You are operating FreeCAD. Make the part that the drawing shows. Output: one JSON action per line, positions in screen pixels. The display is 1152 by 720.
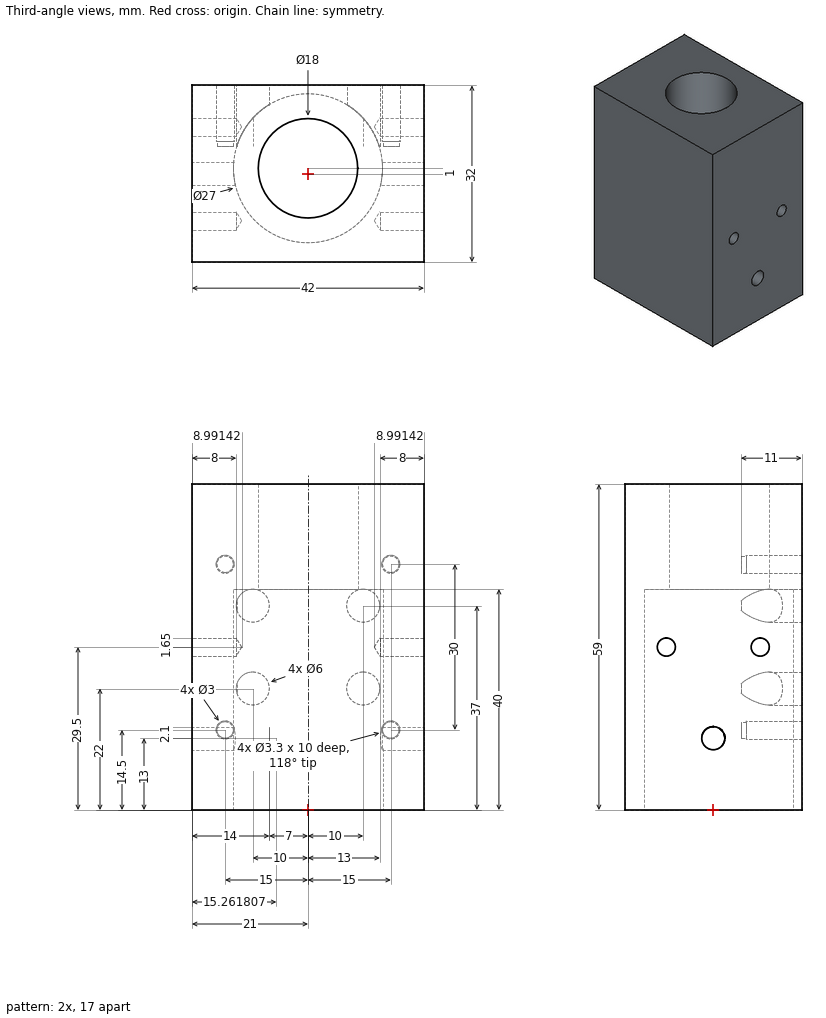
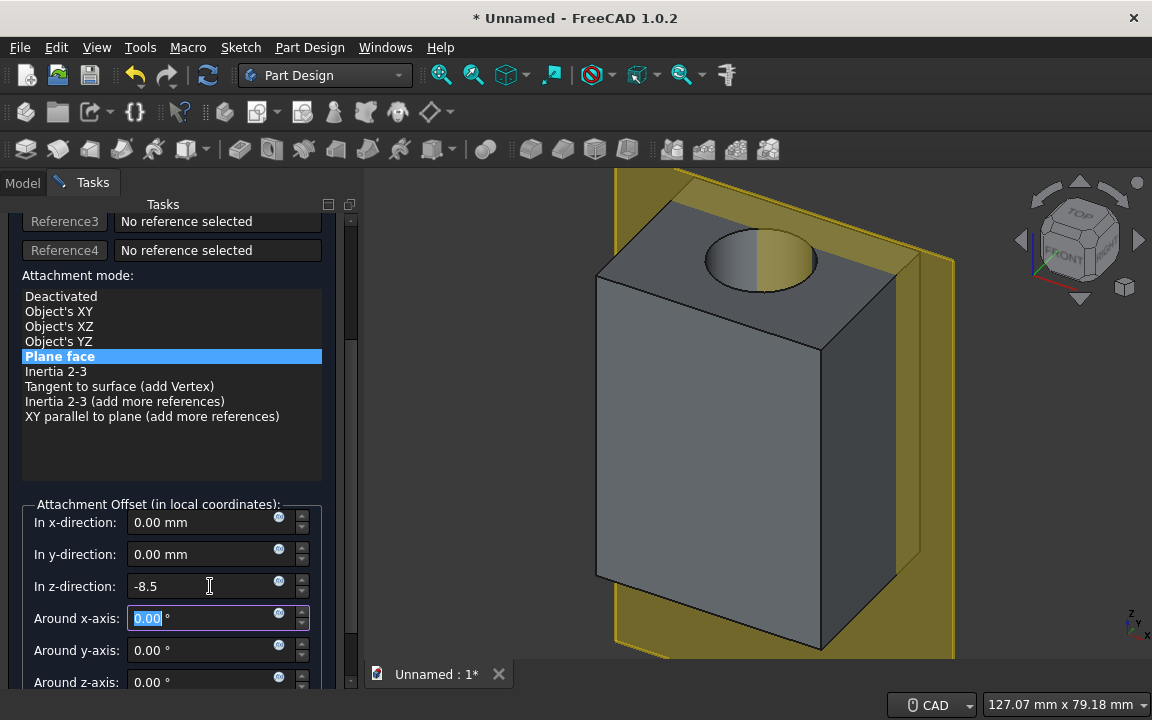
{"action": "scroll", "coordinate": [351, 451], "scroll_direction": "up", "scroll_amount": 4}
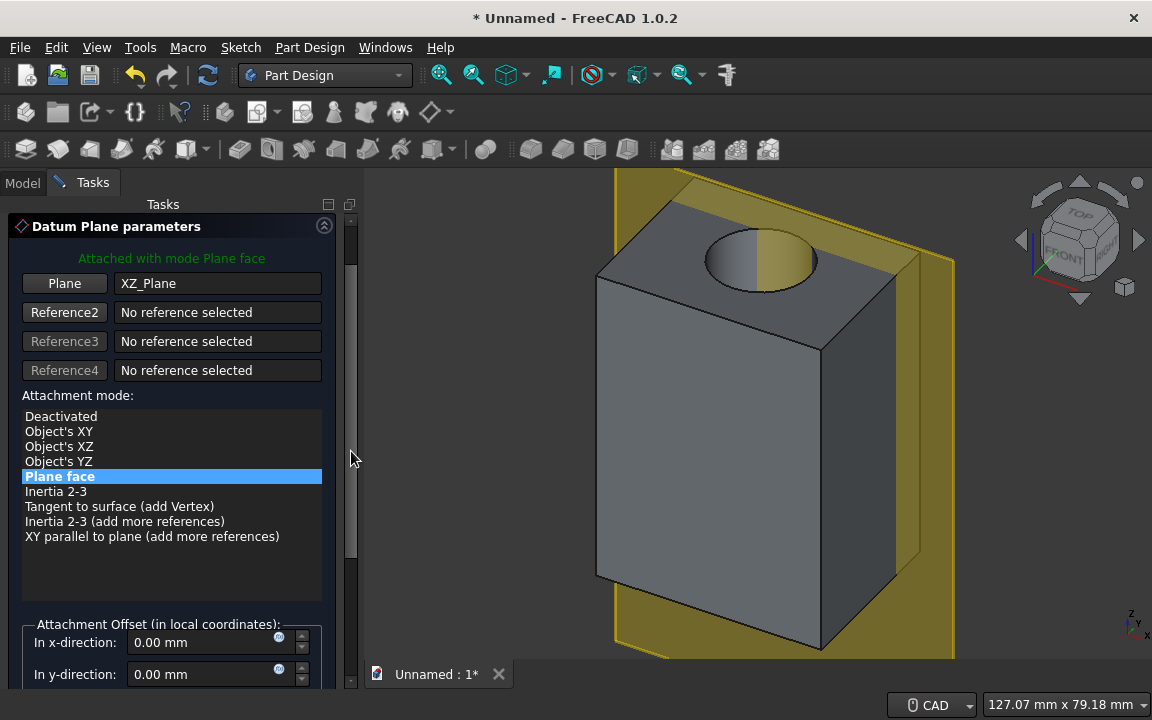
{"action": "left_click", "coordinate": [124, 243]}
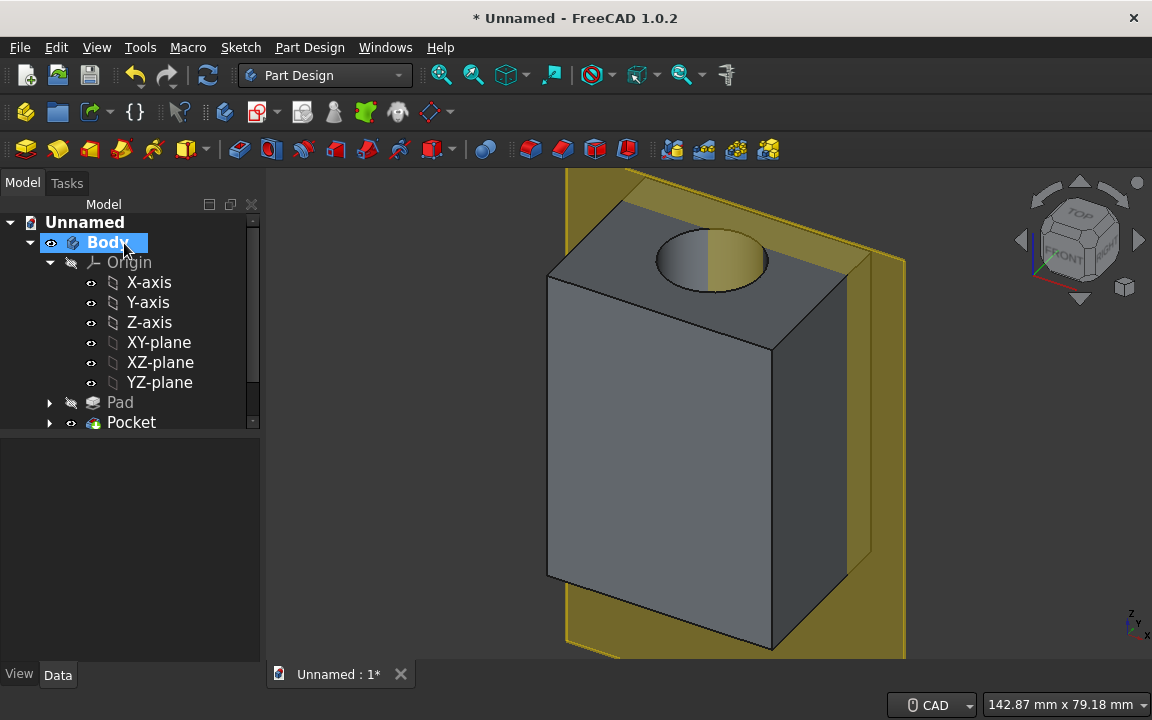
{"action": "scroll", "coordinate": [100, 318], "scroll_direction": "down", "scroll_amount": 3}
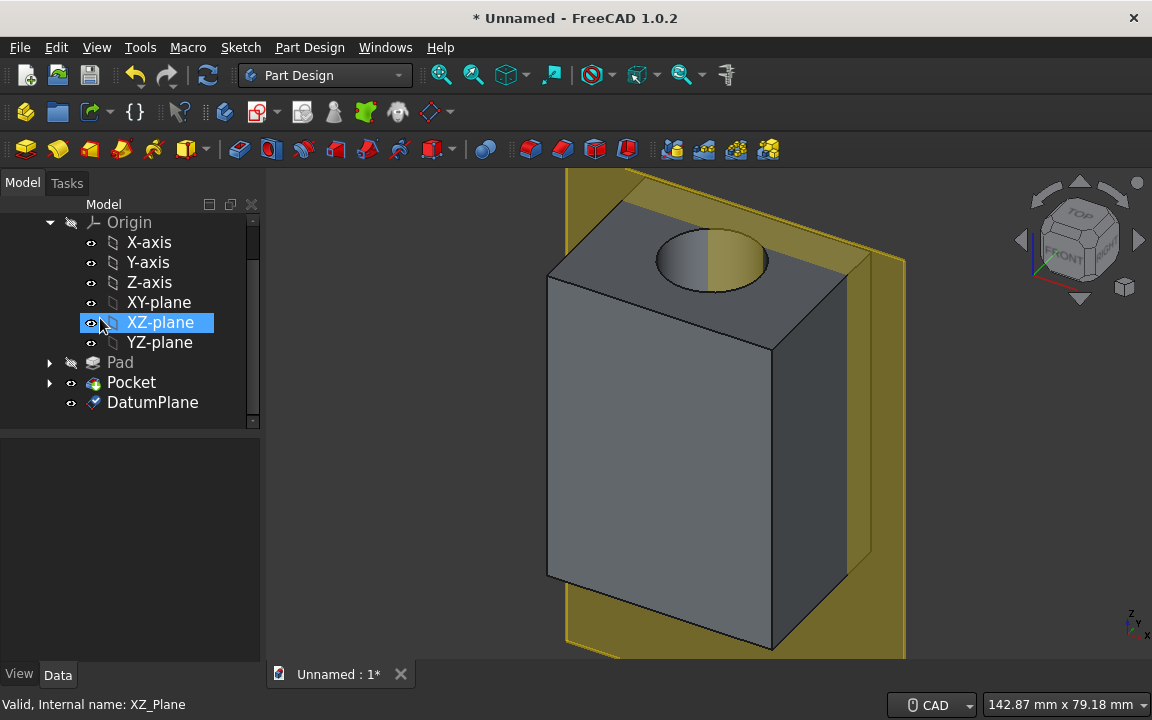
{"action": "left_click", "coordinate": [116, 403]}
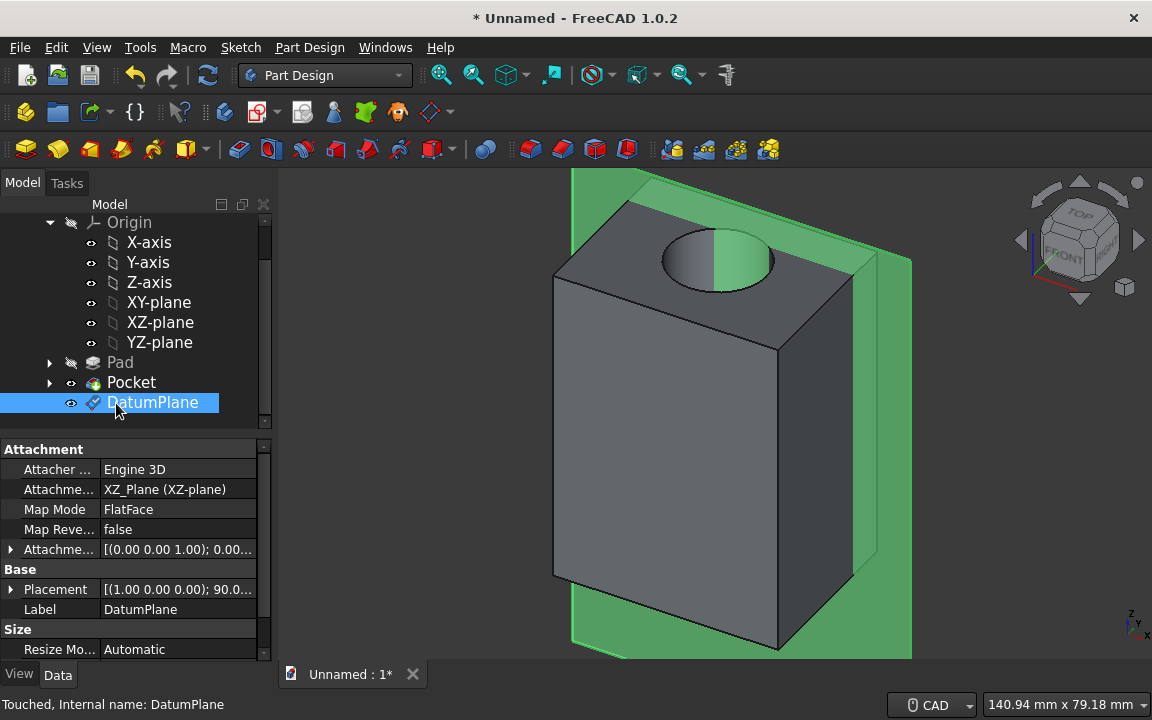
{"action": "left_click", "coordinate": [258, 112]}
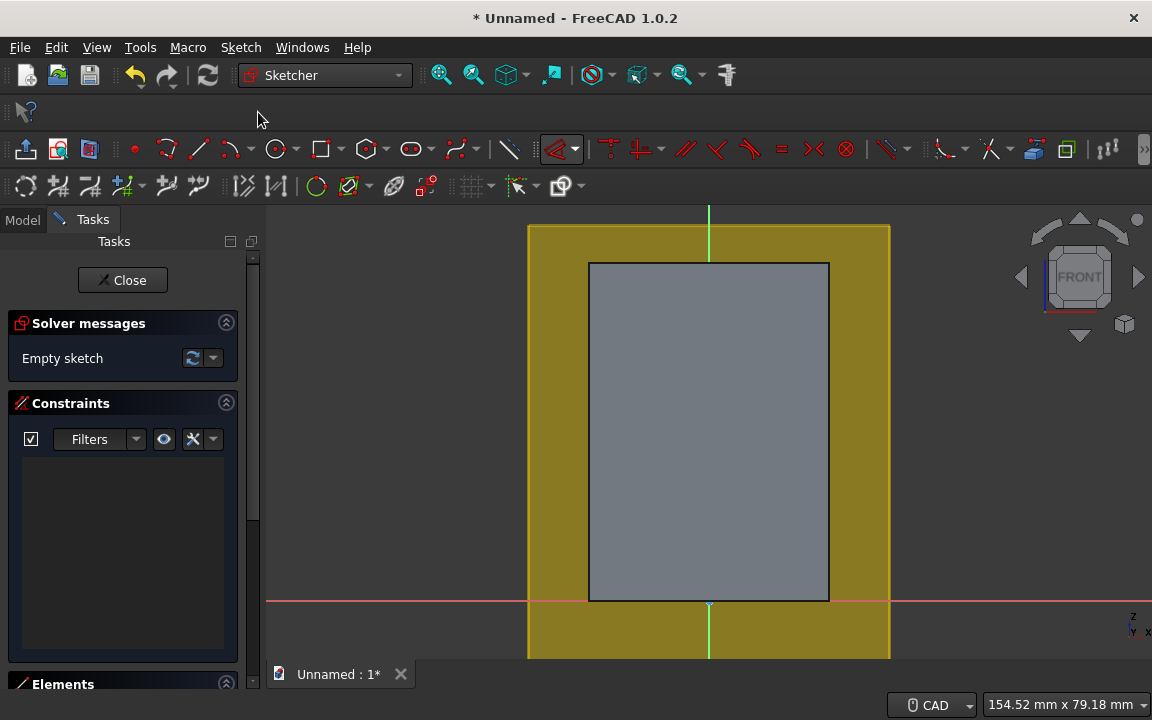
{"action": "key", "text": "q s"}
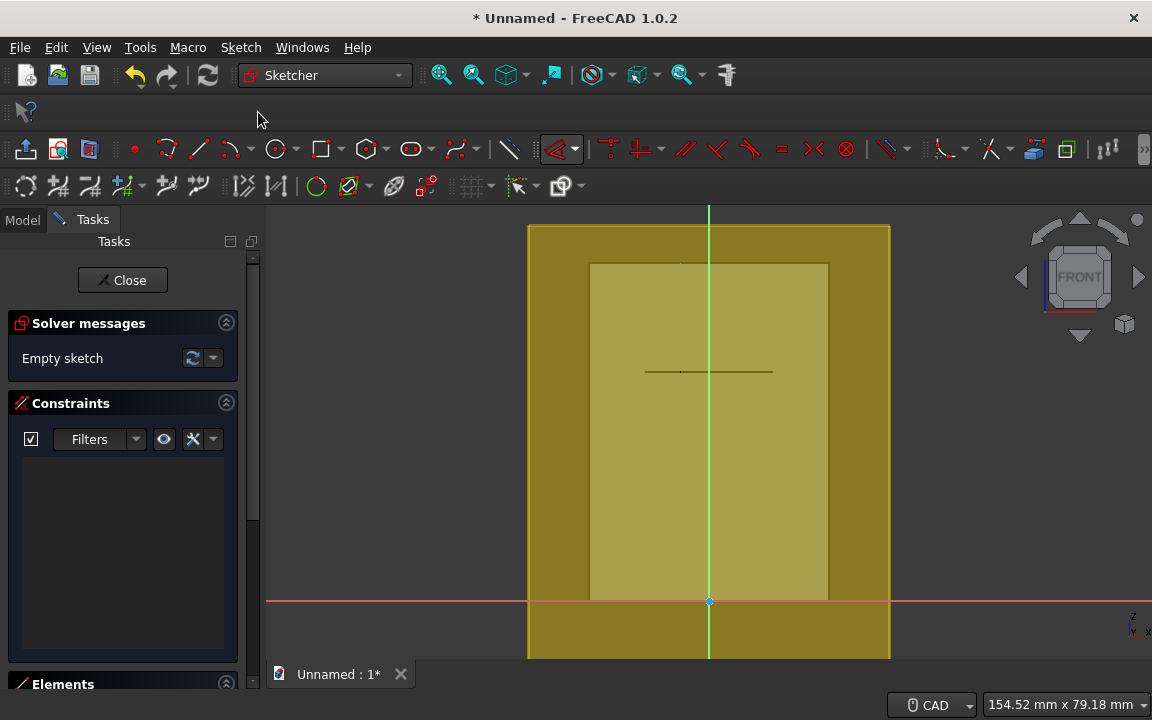
{"action": "scroll", "coordinate": [666, 631], "scroll_direction": "up", "scroll_amount": 2}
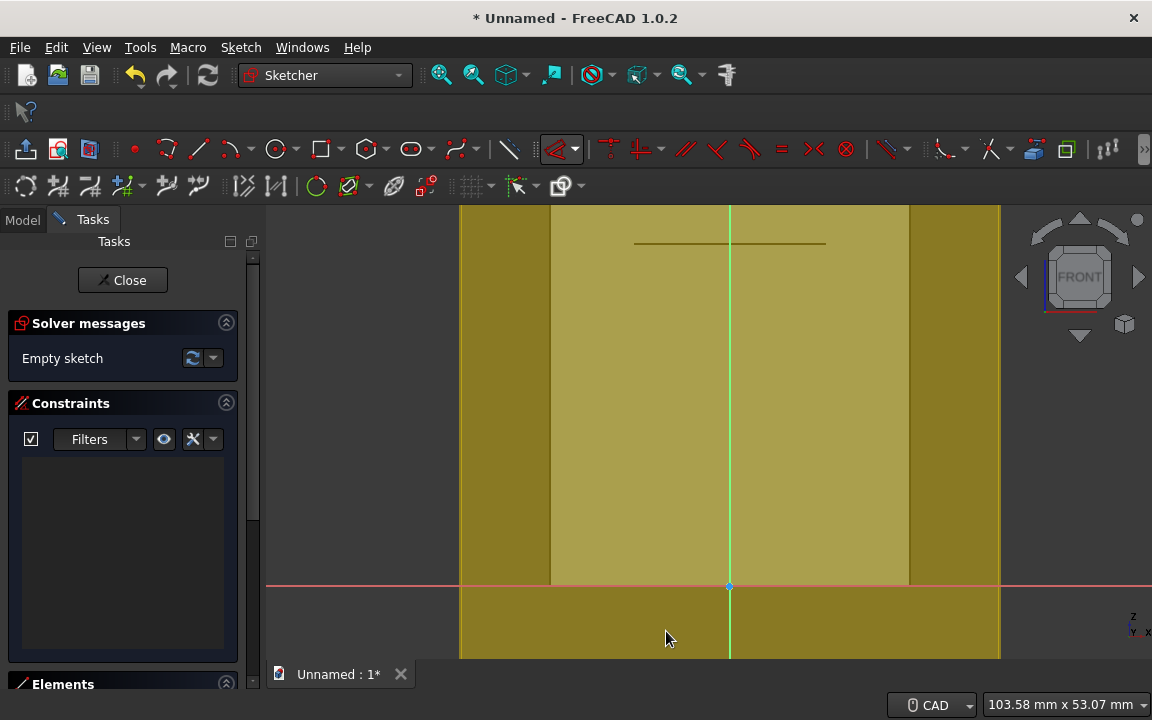
{"action": "key", "text": "g m"}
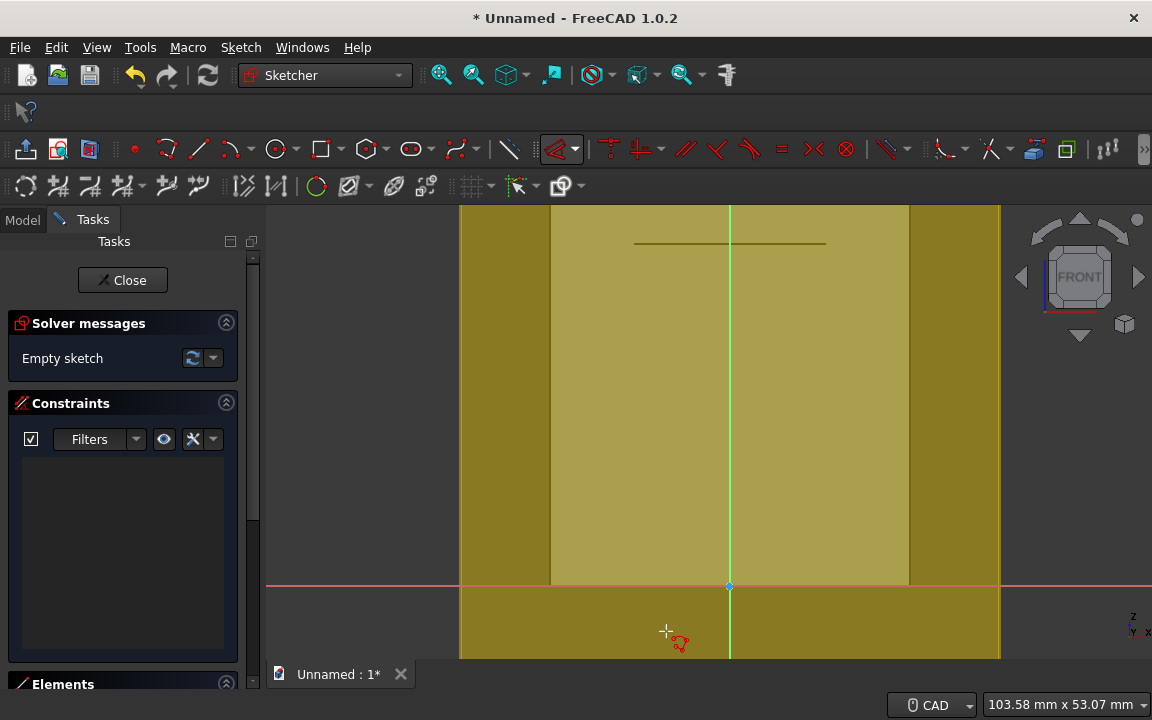
{"action": "left_click", "coordinate": [627, 334]}
{"action": "left_click", "coordinate": [550, 334]}
{"action": "left_click", "coordinate": [550, 320]}
{"action": "left_click", "coordinate": [619, 320]}
{"action": "left_click", "coordinate": [627, 335]}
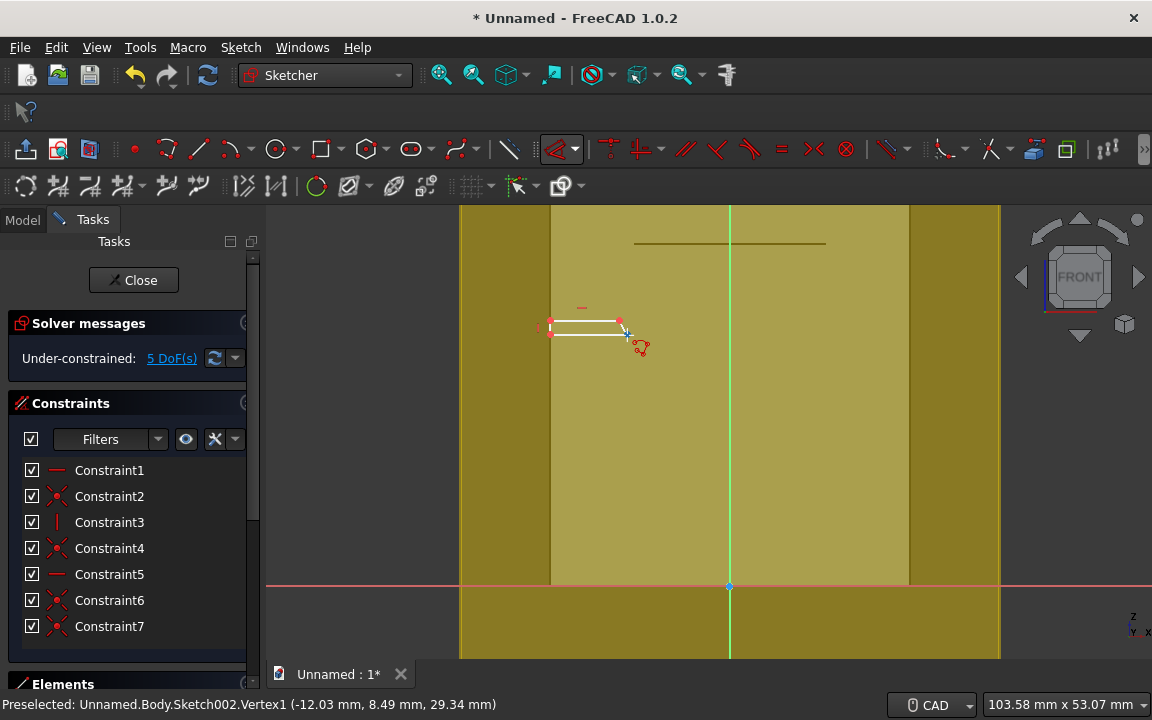
{"action": "left_click", "coordinate": [200, 150]}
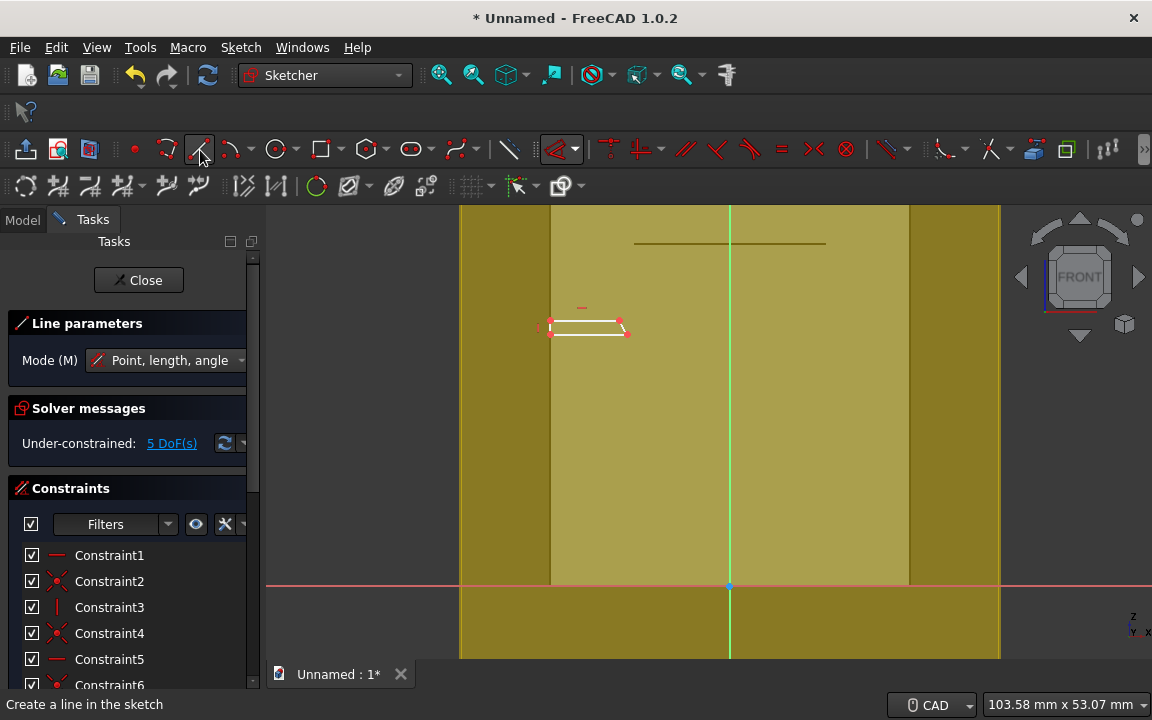
{"action": "scroll", "coordinate": [635, 334], "scroll_direction": "up", "scroll_amount": 4}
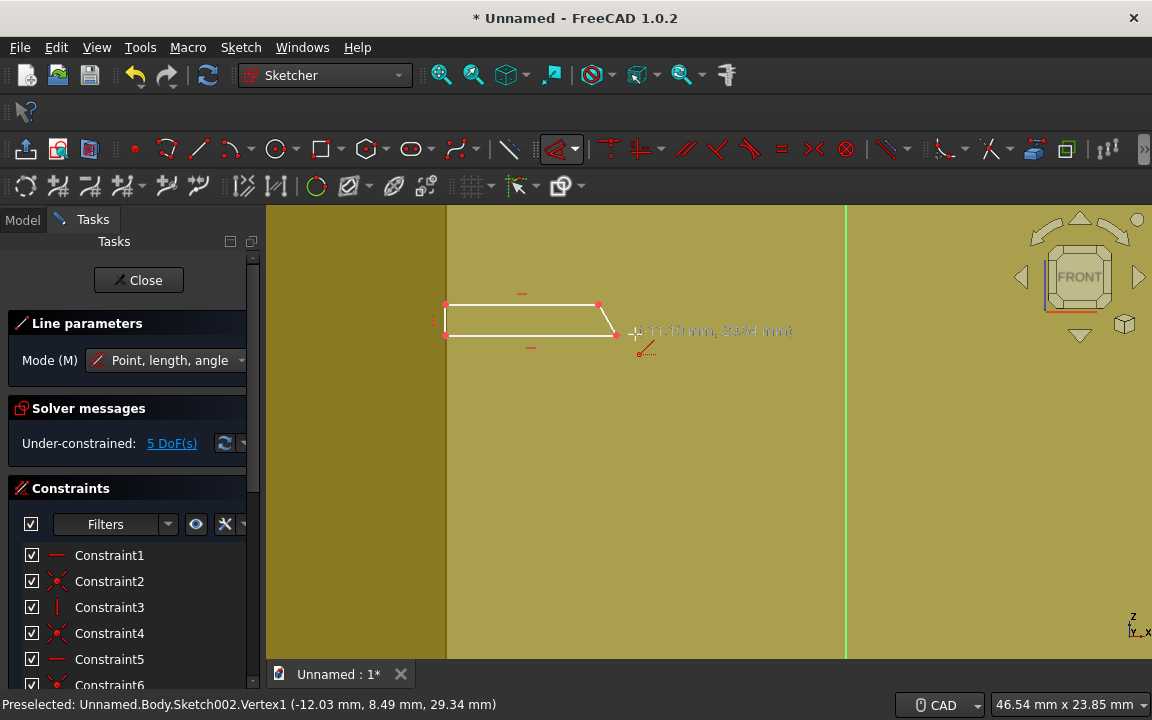
{"action": "left_click", "coordinate": [634, 333]}
{"action": "left_click", "coordinate": [686, 333]}
{"action": "key", "text": "Escape"}